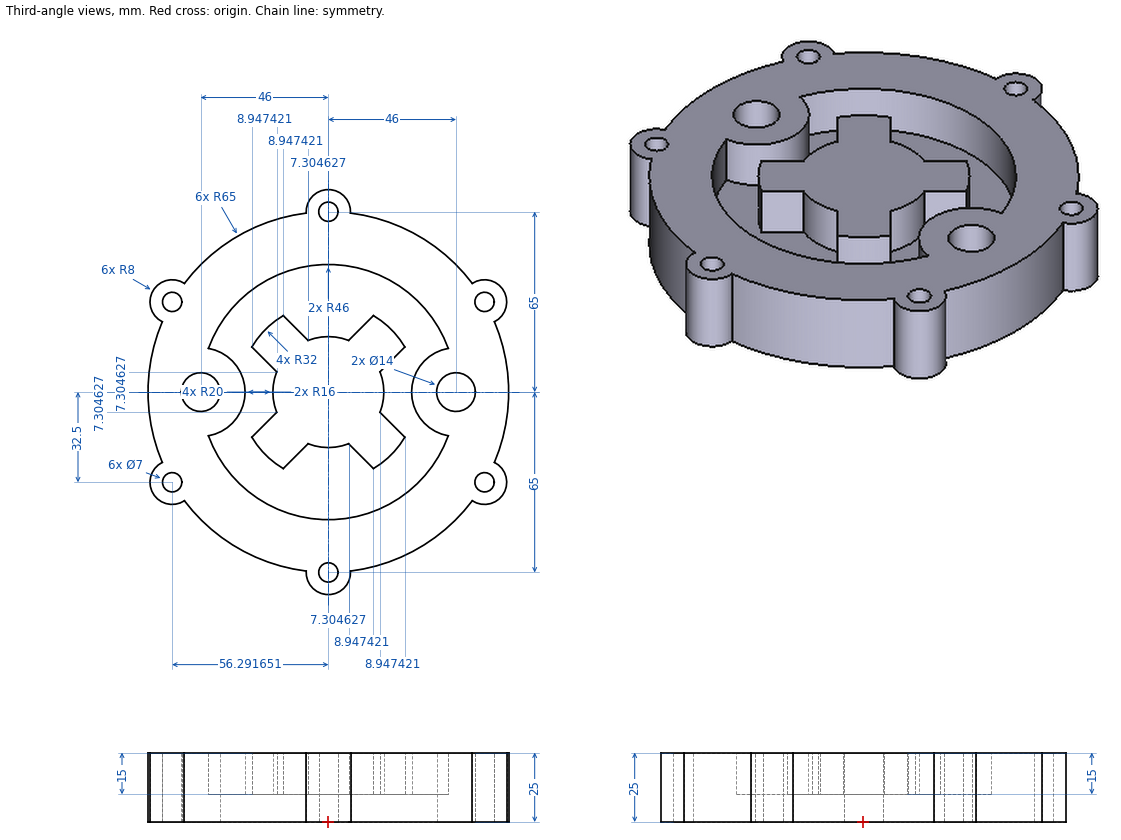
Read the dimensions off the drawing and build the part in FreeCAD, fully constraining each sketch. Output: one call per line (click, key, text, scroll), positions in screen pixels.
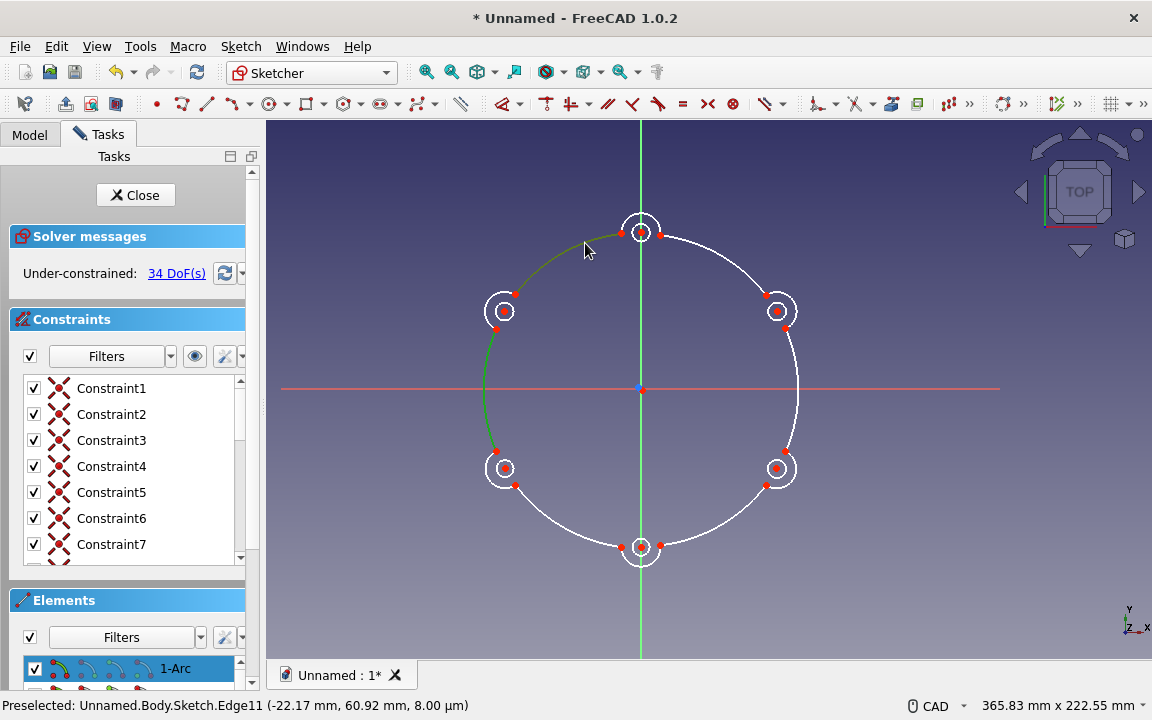
click(546, 104)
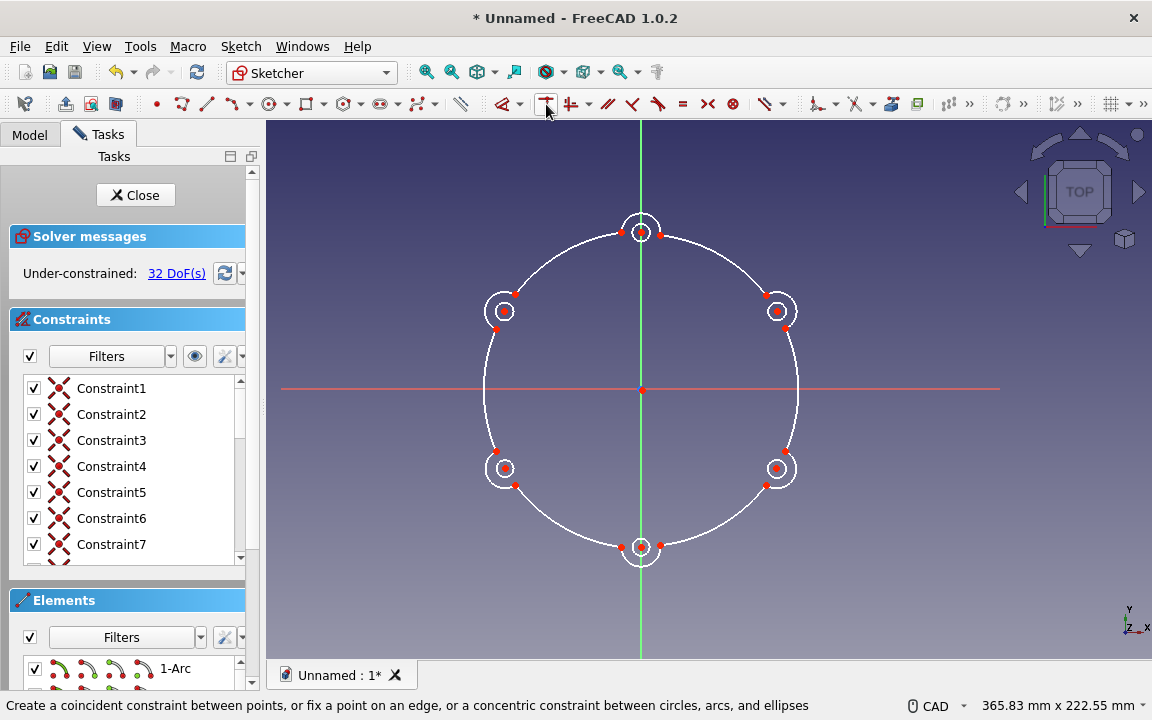
scroll(642, 390, up, 8)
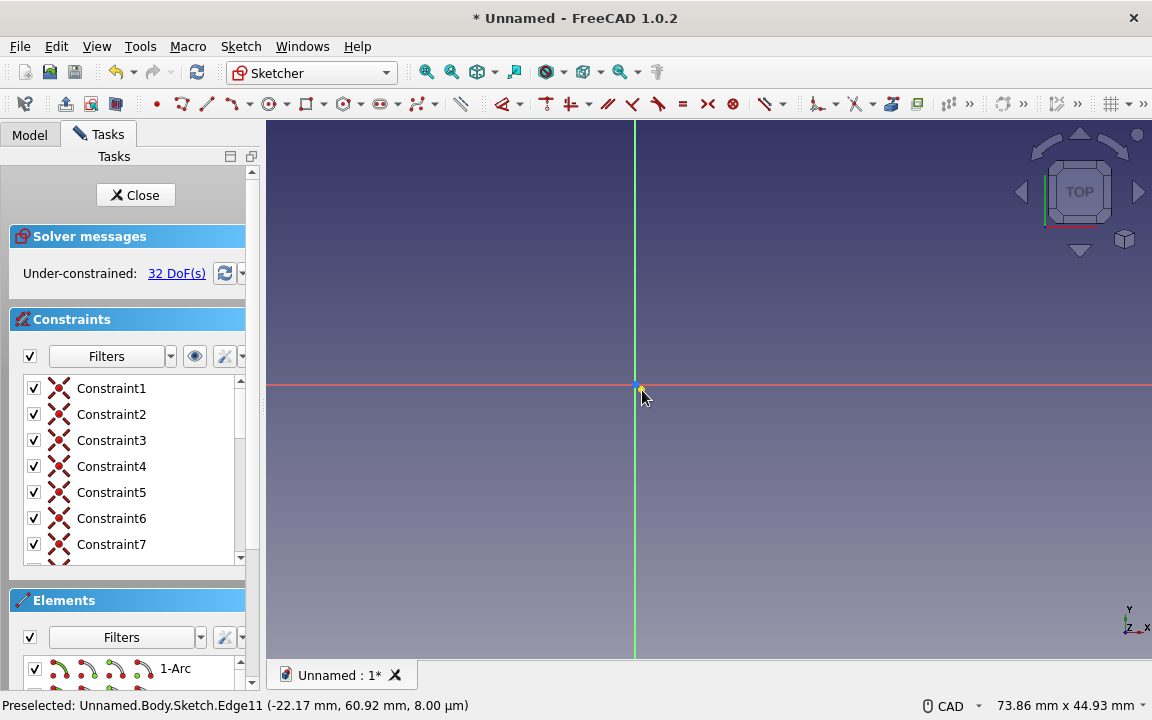
drag(625, 375, 652, 399)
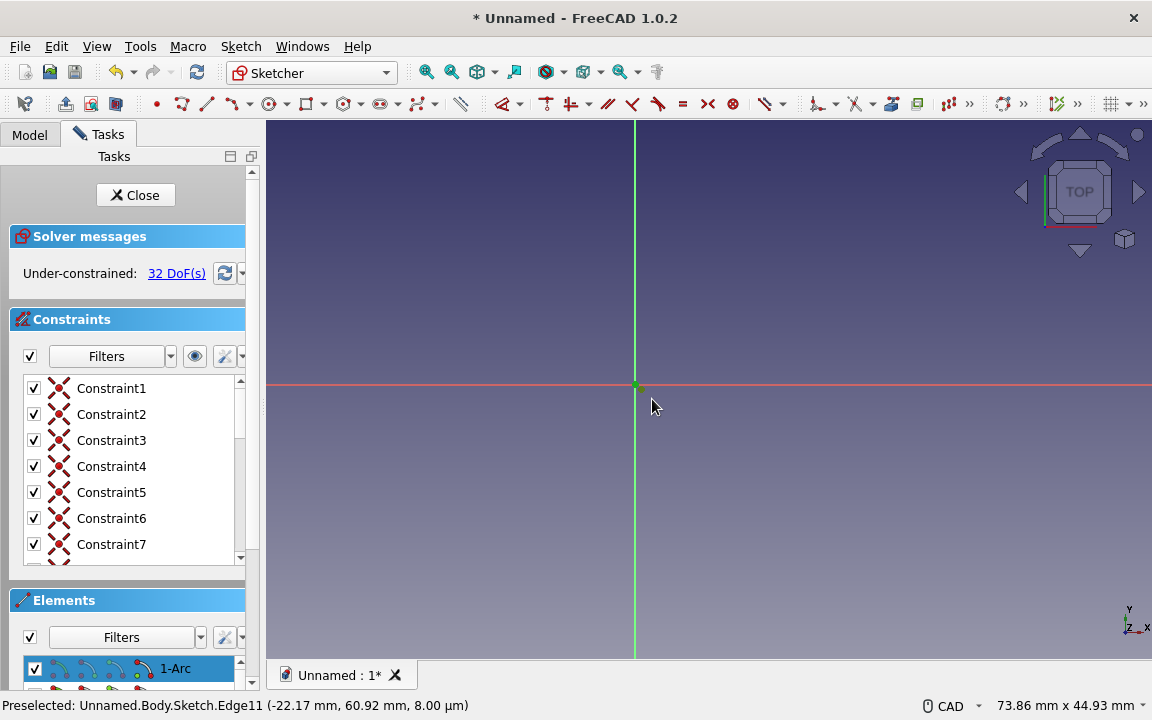
click(546, 104)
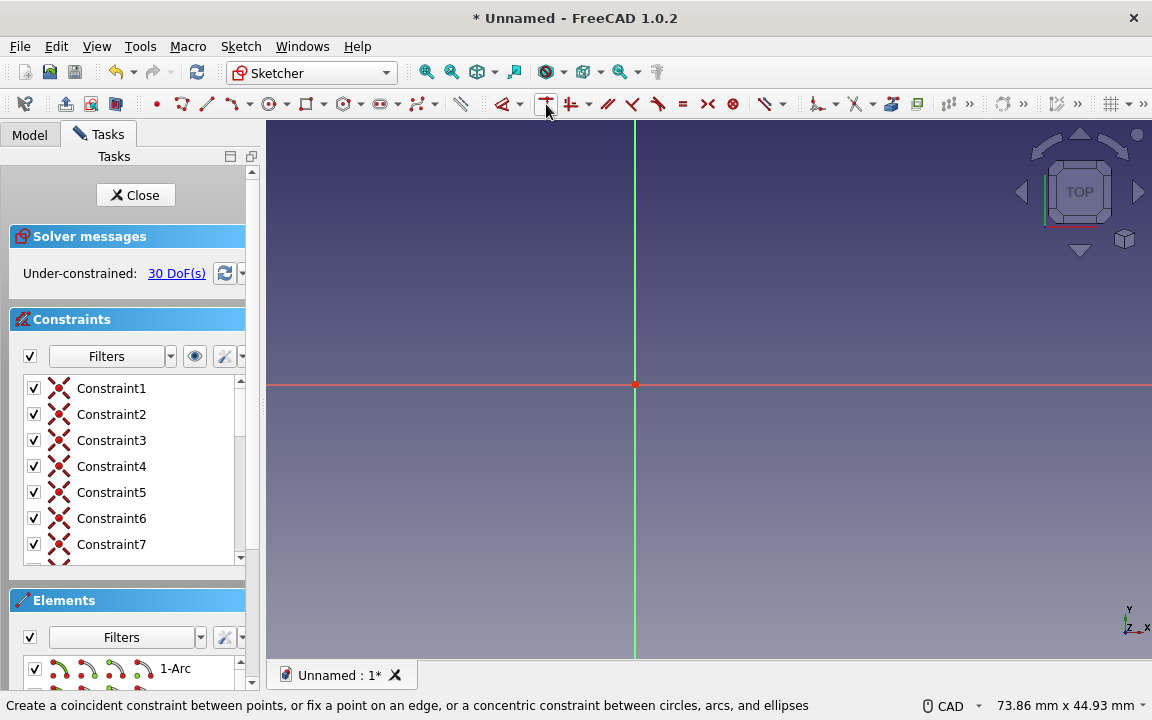
scroll(642, 391, down, 8)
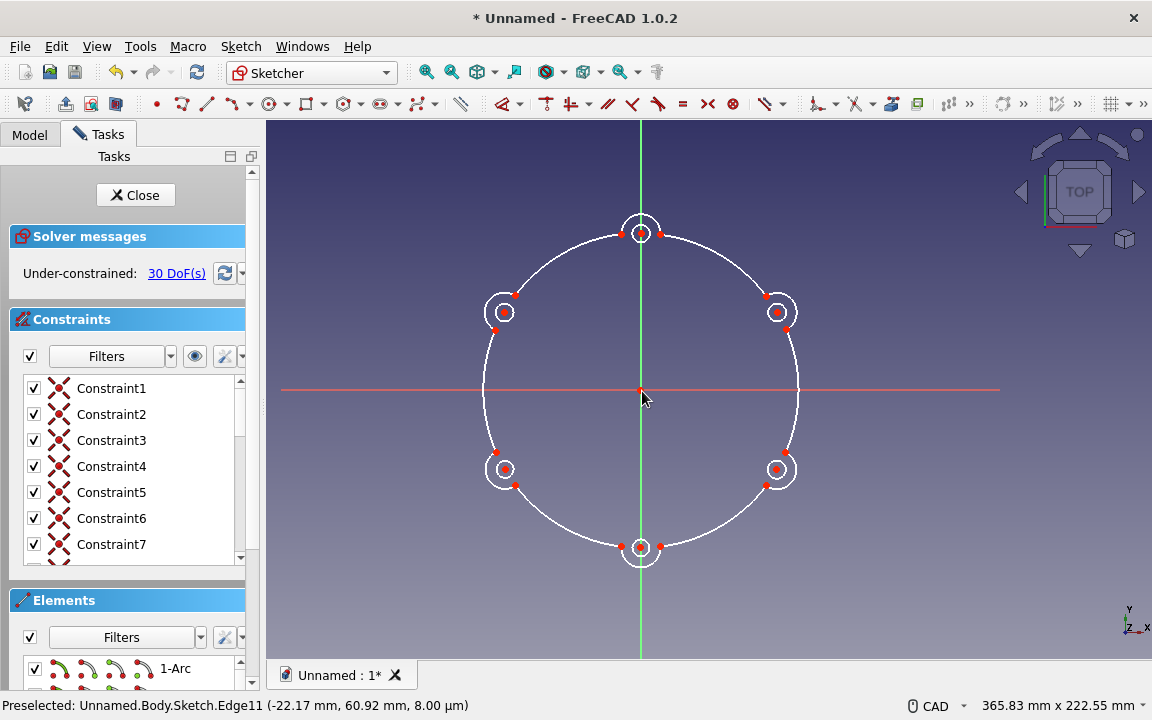
click(485, 366)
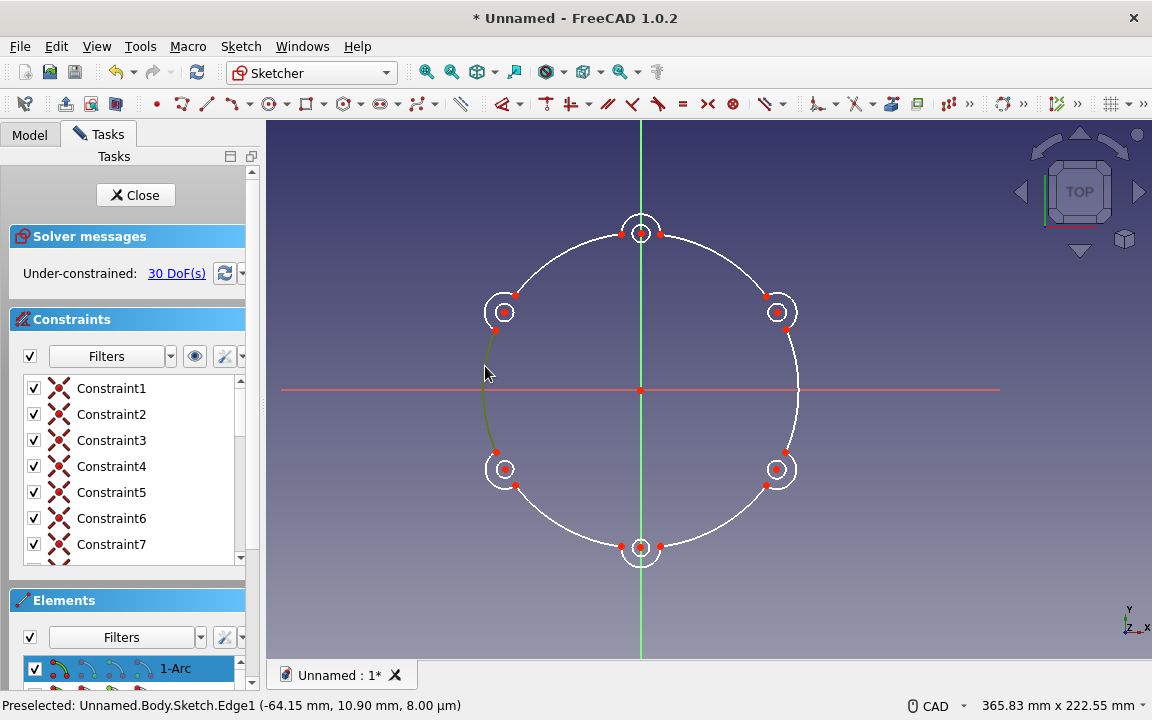
click(542, 513)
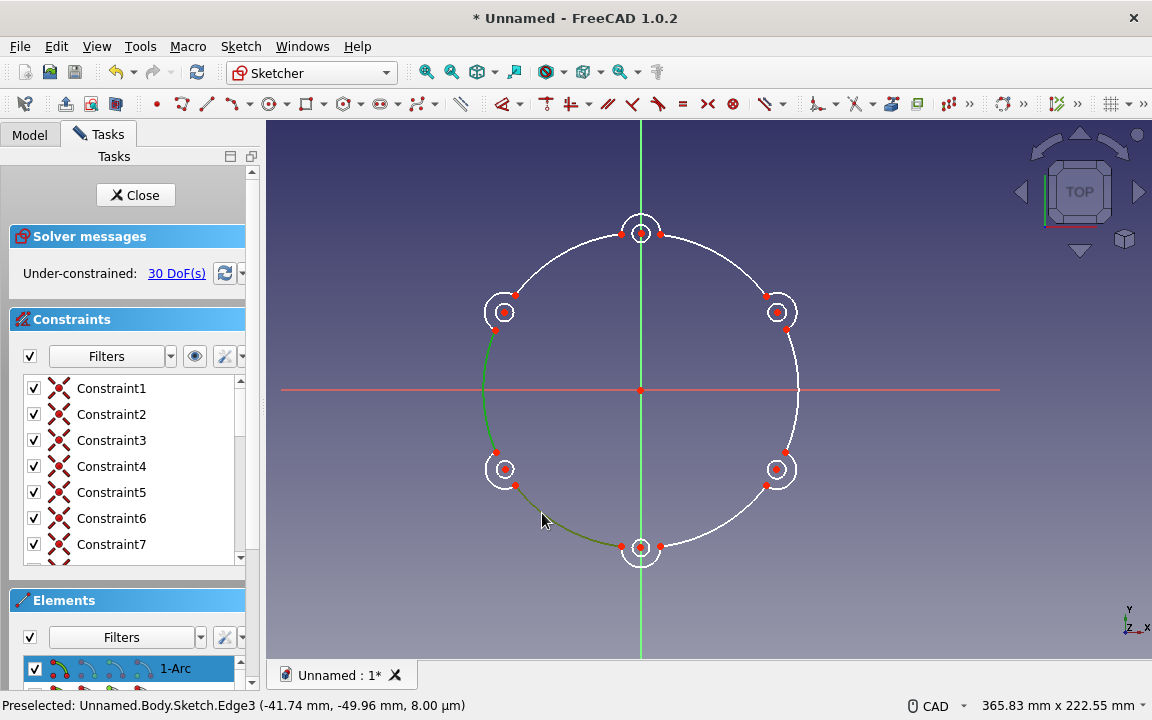
click(697, 538)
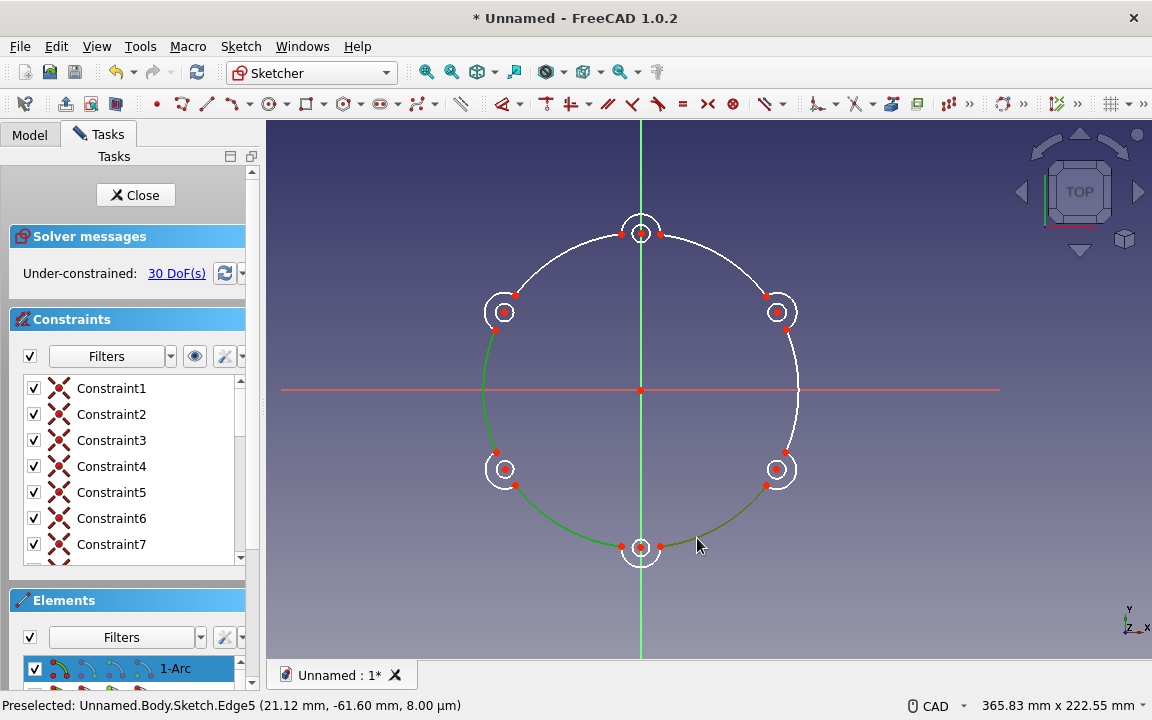
click(796, 416)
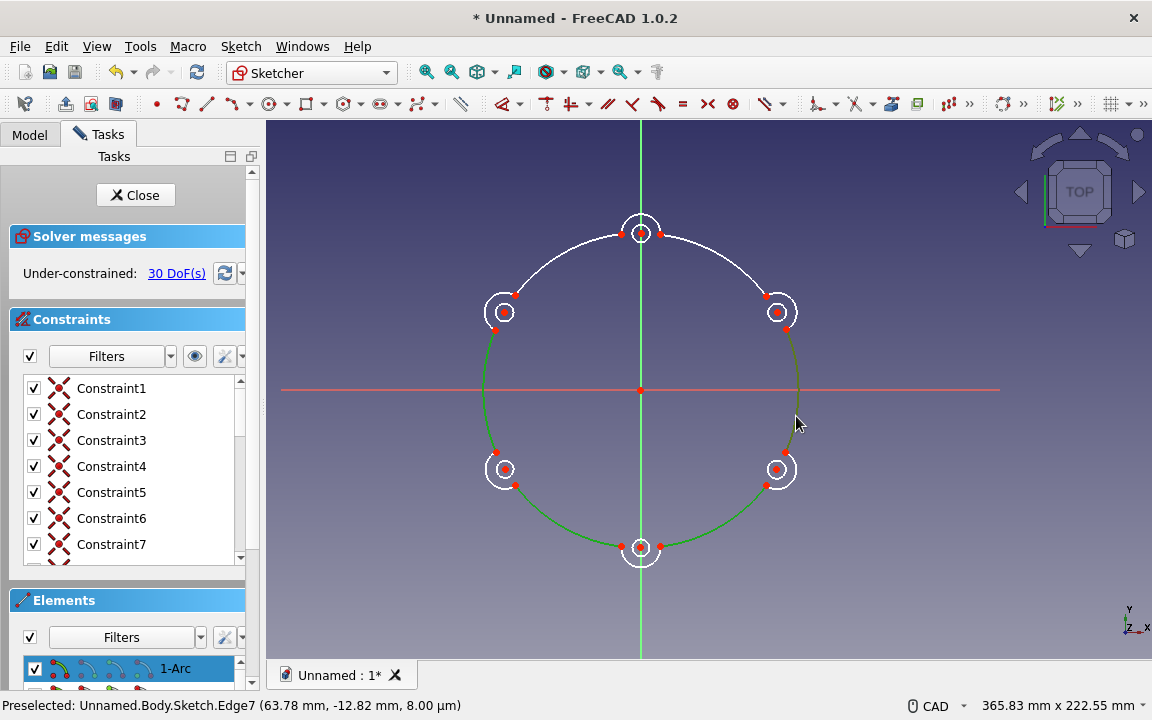
click(740, 269)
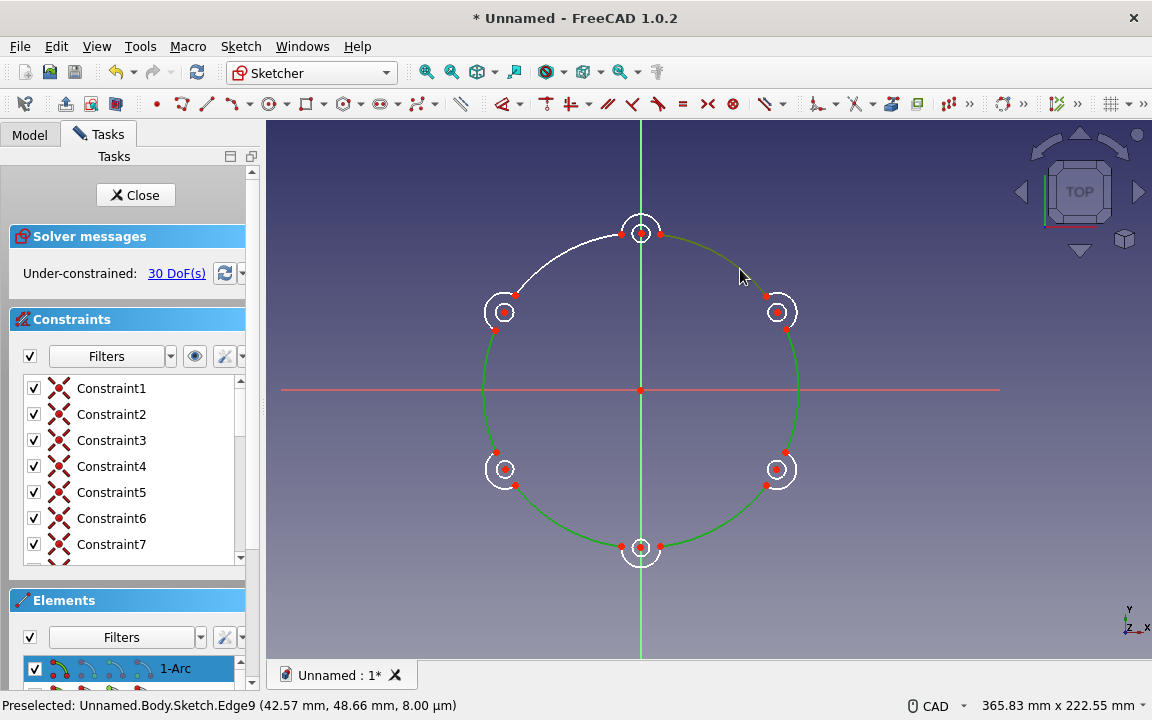
click(585, 243)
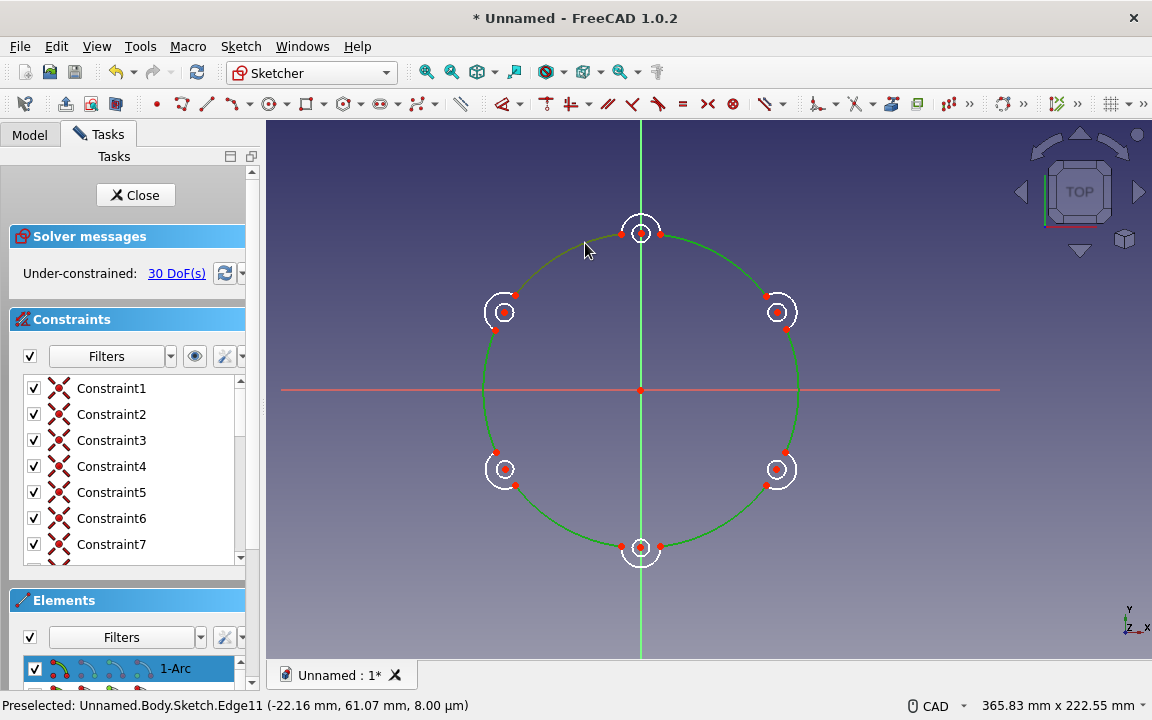
click(683, 104)